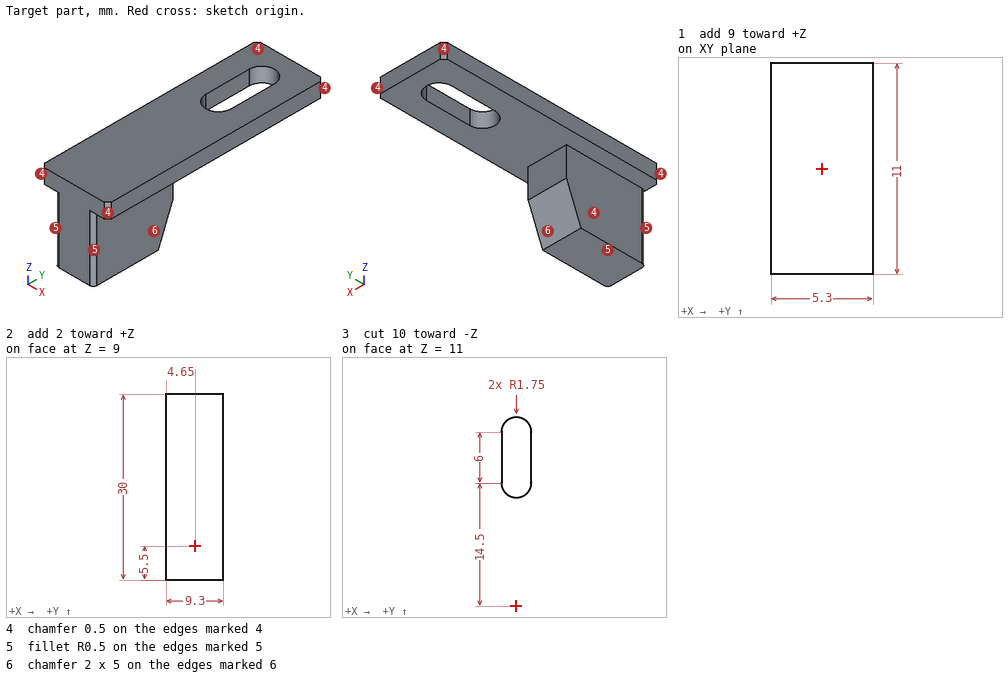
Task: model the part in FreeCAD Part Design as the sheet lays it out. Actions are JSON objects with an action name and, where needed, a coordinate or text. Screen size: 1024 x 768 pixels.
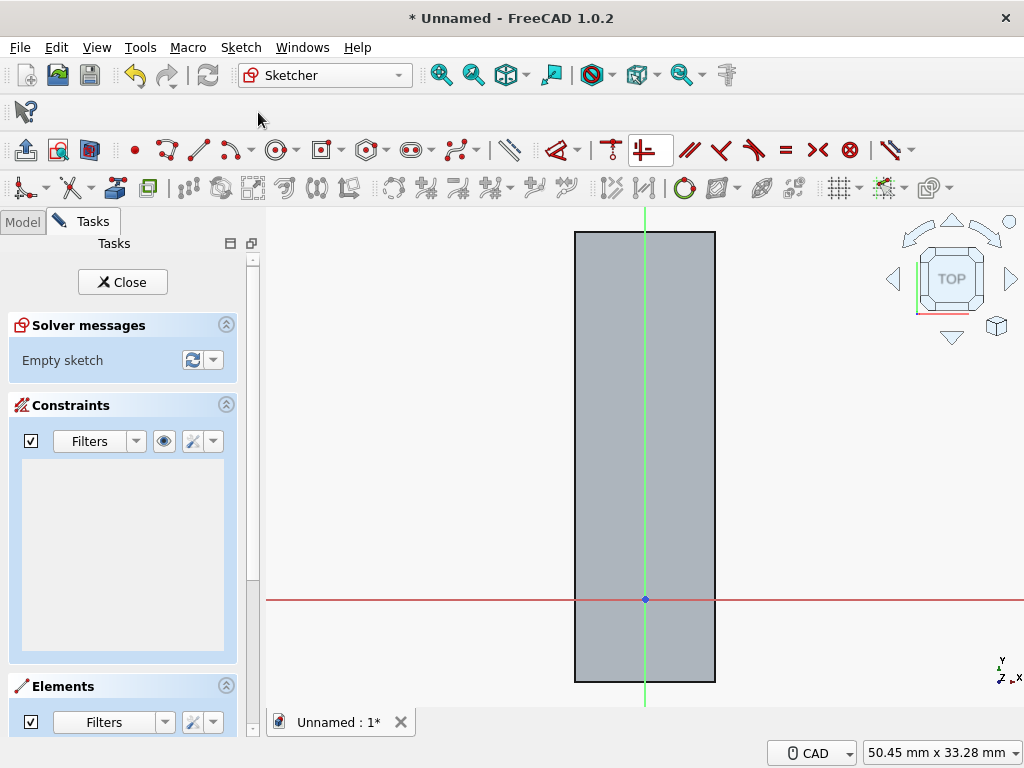
{"action": "left_click", "coordinate": [645, 382]}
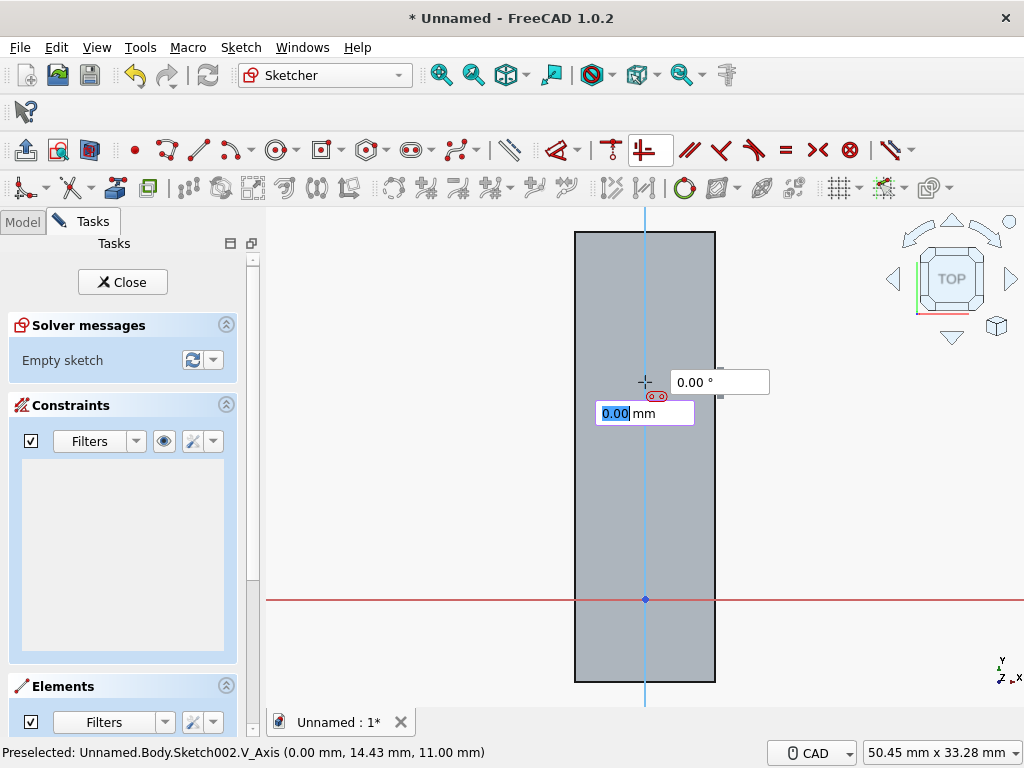
{"action": "left_click", "coordinate": [654, 292]}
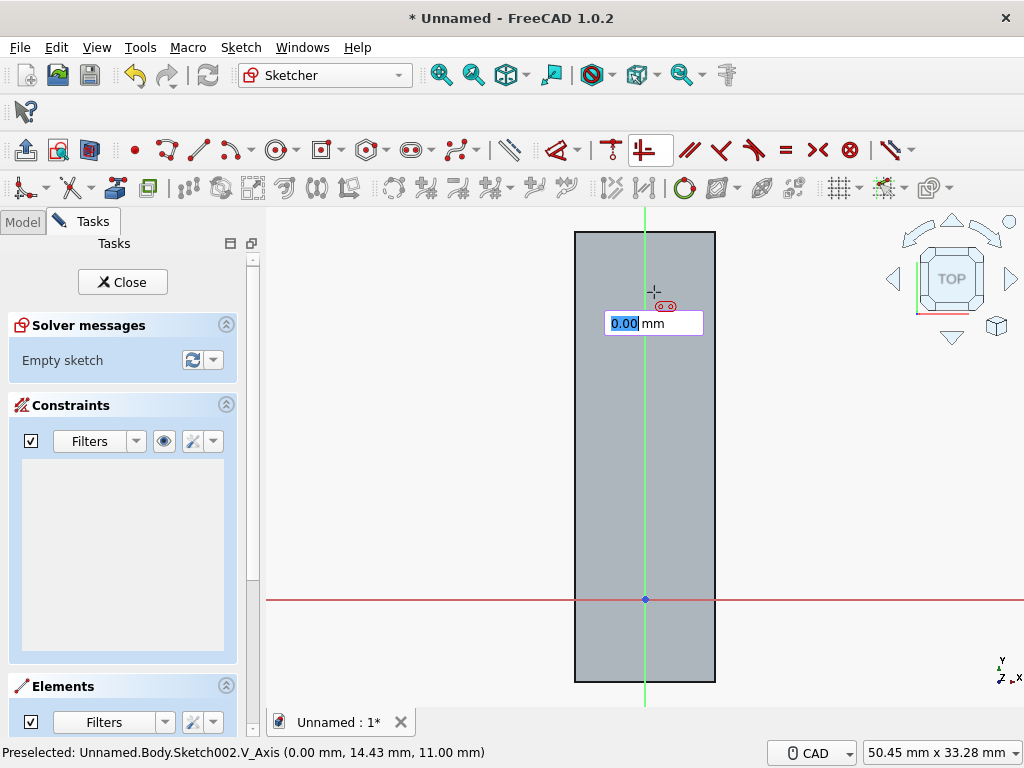
{"action": "left_click", "coordinate": [671, 337]}
{"action": "key", "text": "Escape"}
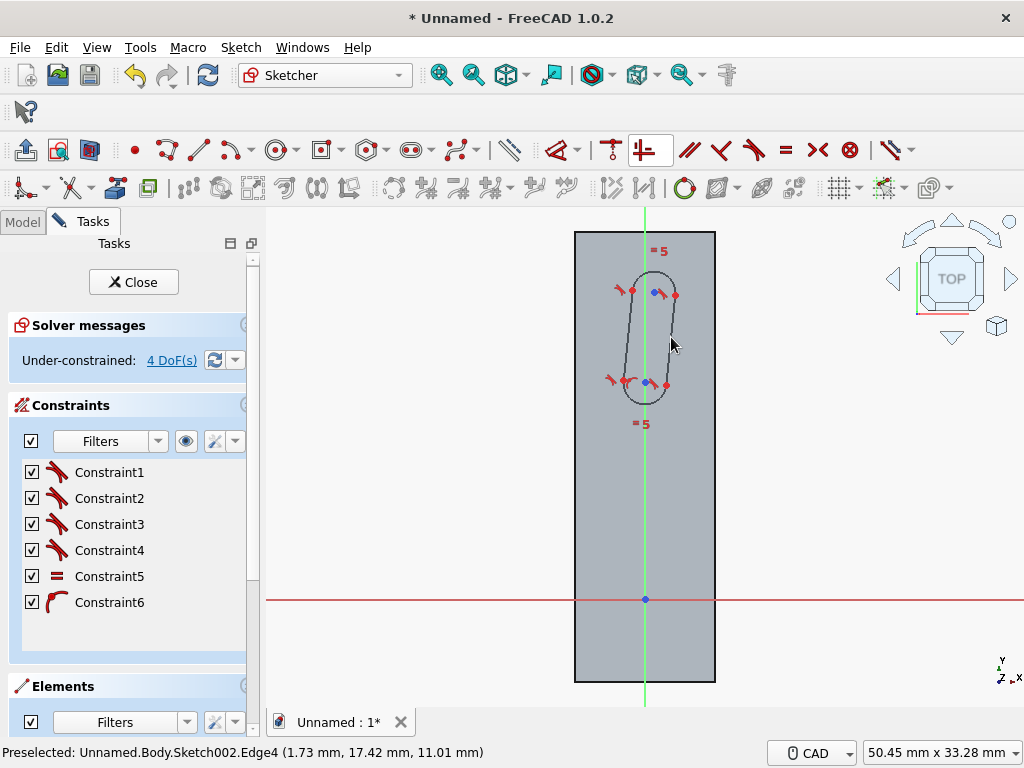
{"action": "left_click", "coordinate": [626, 354]}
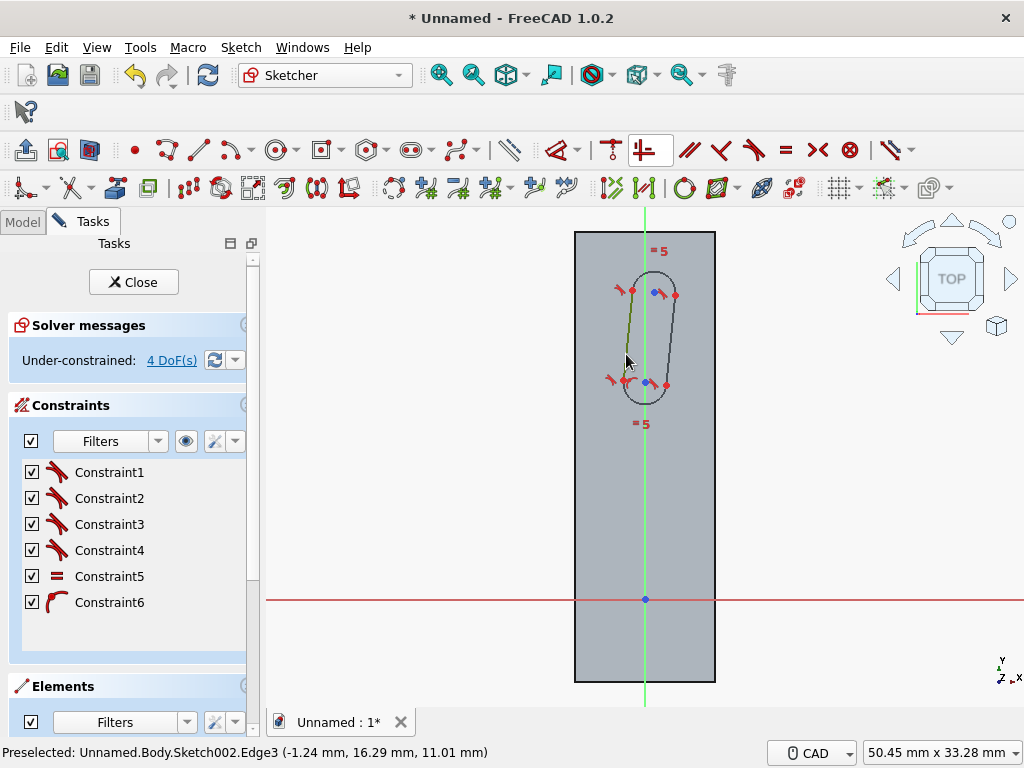
{"action": "key", "text": "v"}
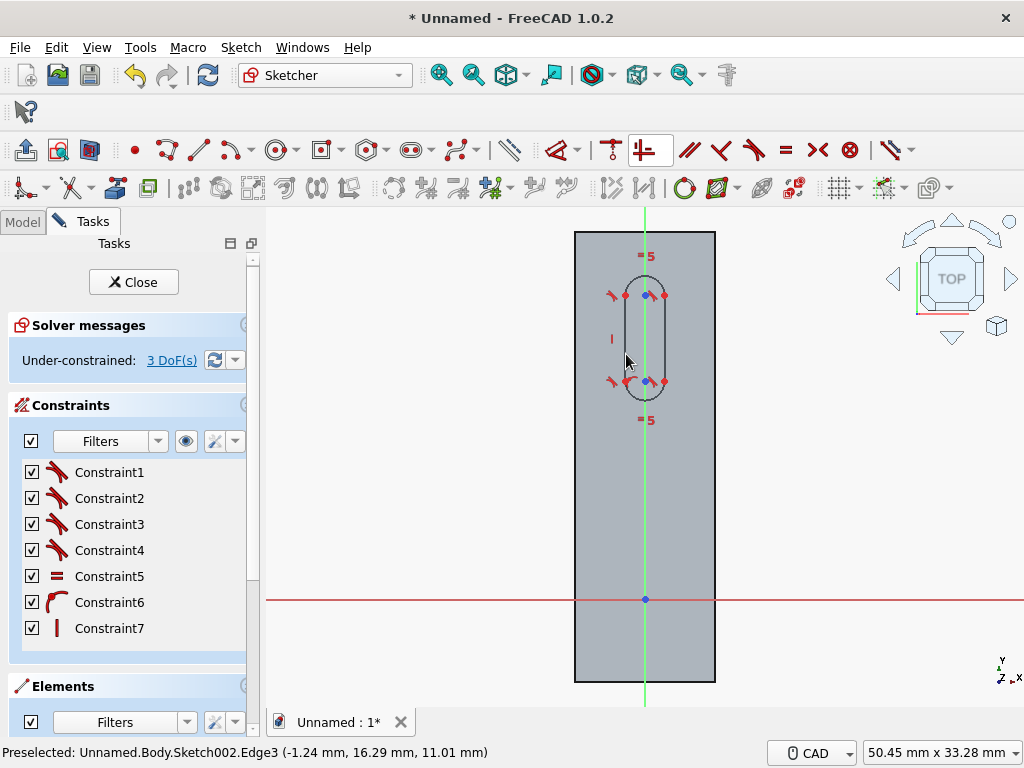
{"action": "left_click", "coordinate": [556, 150]}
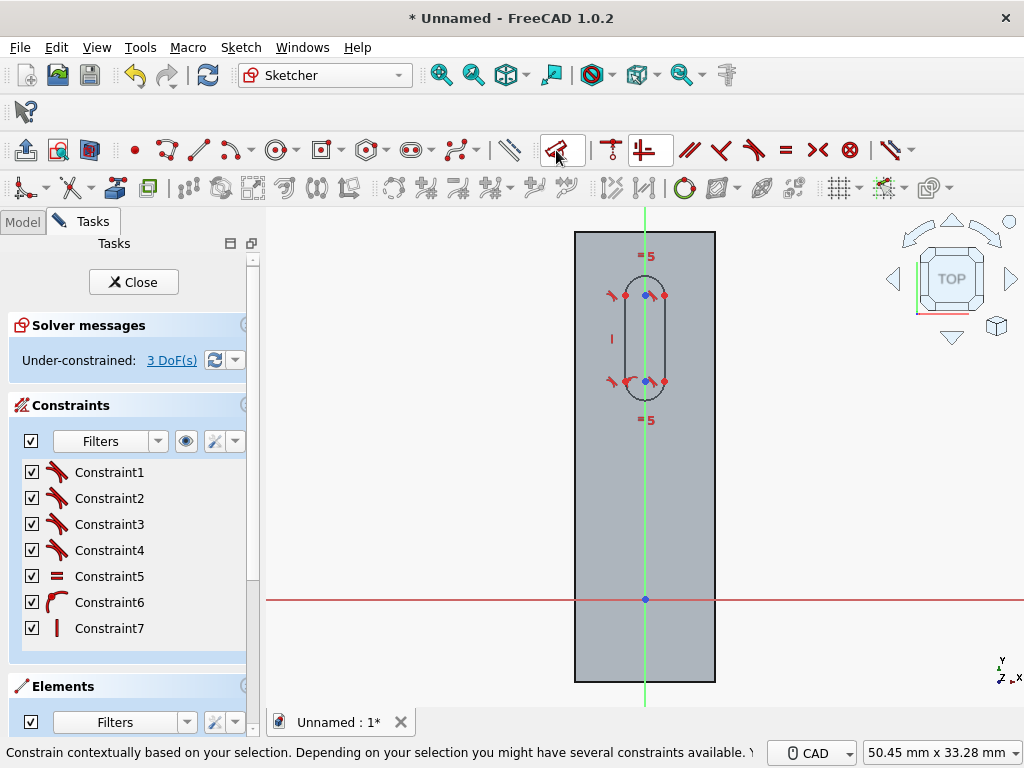
{"action": "scroll", "coordinate": [634, 397], "scroll_direction": "up", "scroll_amount": 3}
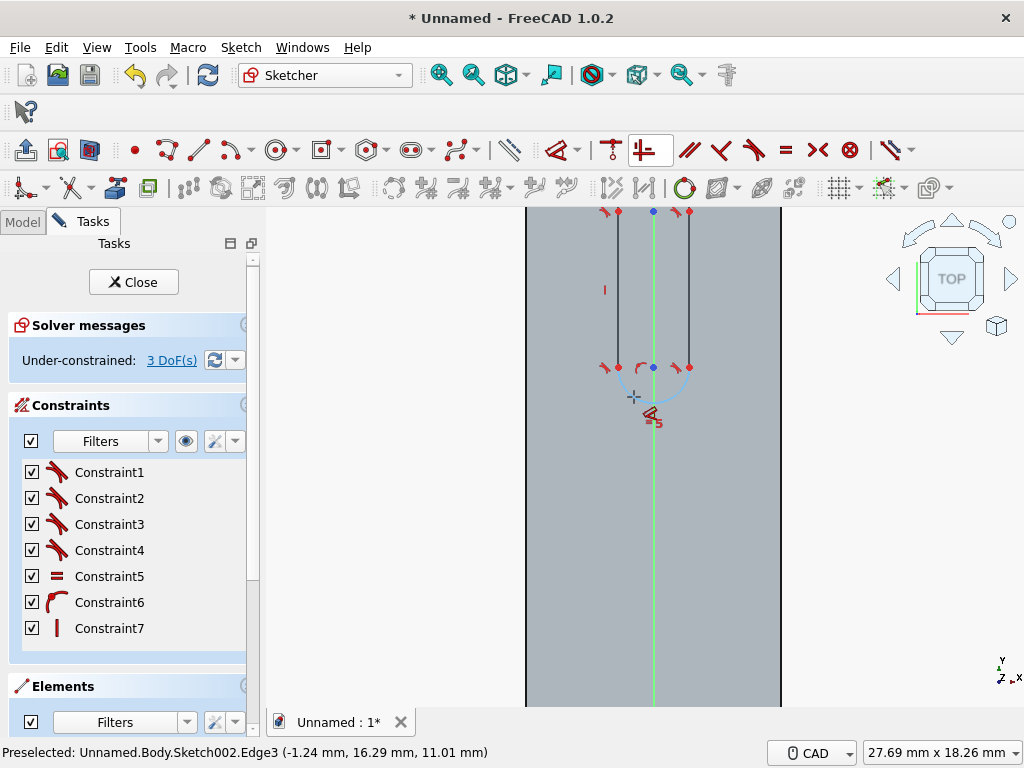
{"action": "left_click", "coordinate": [633, 396]}
{"action": "left_click", "coordinate": [614, 422]}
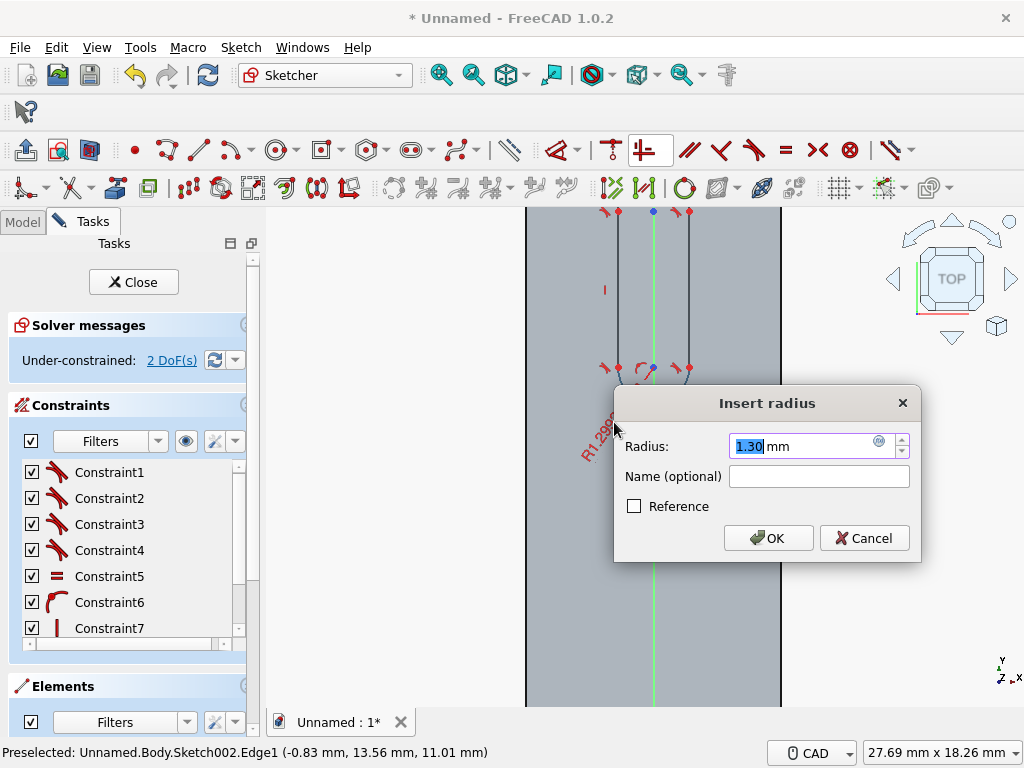
{"action": "type", "text": "1.75"}
{"action": "key", "text": "Return"}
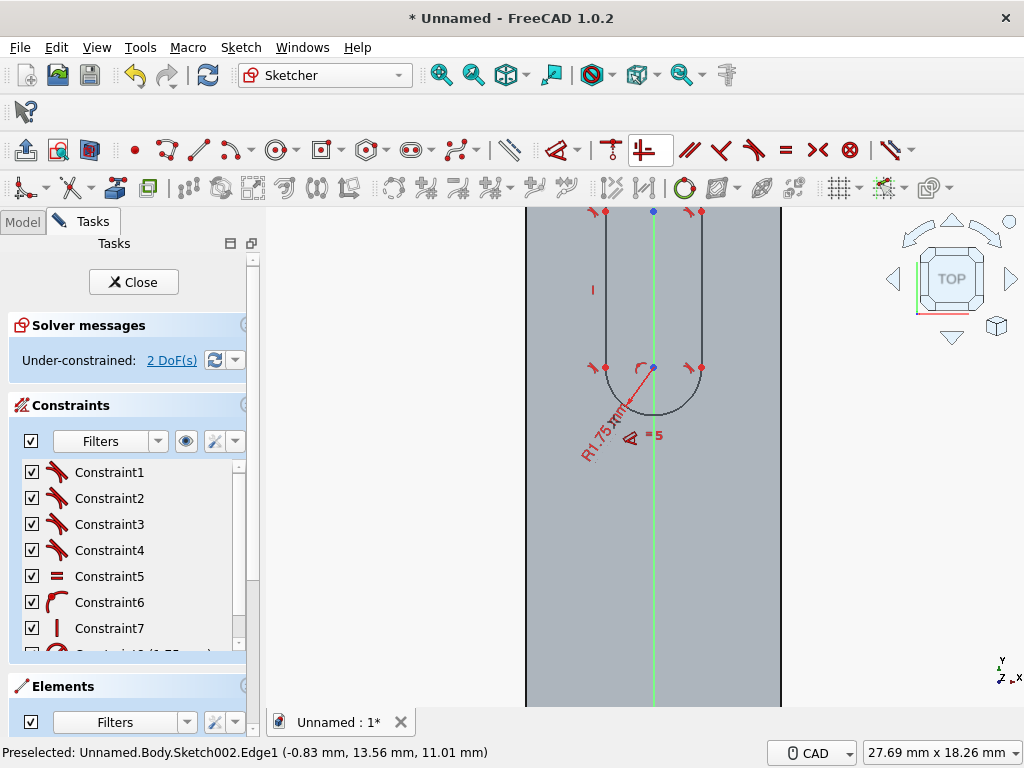
{"action": "left_click", "coordinate": [606, 321]}
{"action": "left_click", "coordinate": [572, 301]}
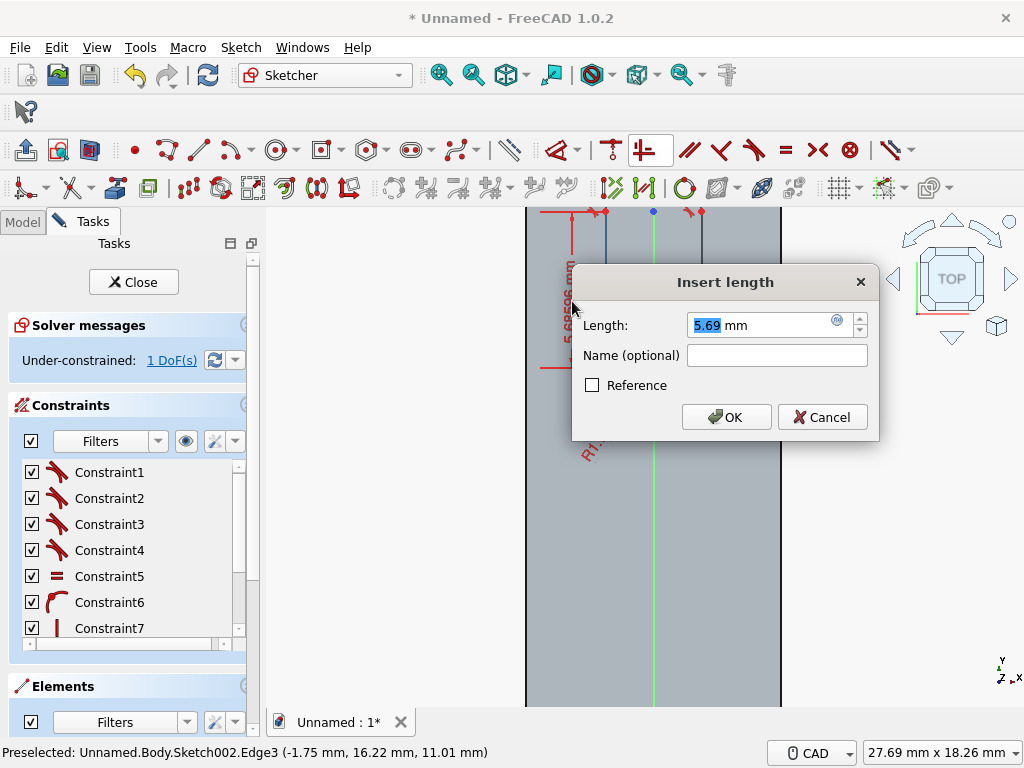
{"action": "type", "text": "6"}
{"action": "key", "text": "Return"}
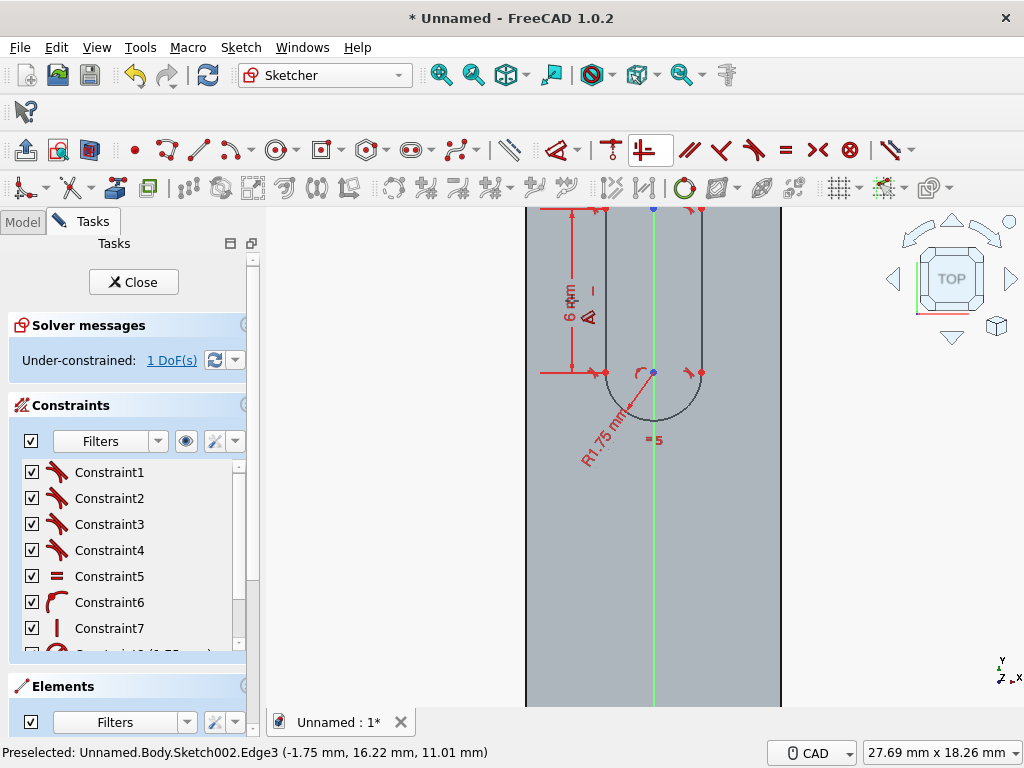
{"action": "left_click", "coordinate": [606, 373]}
{"action": "left_click", "coordinate": [572, 526]}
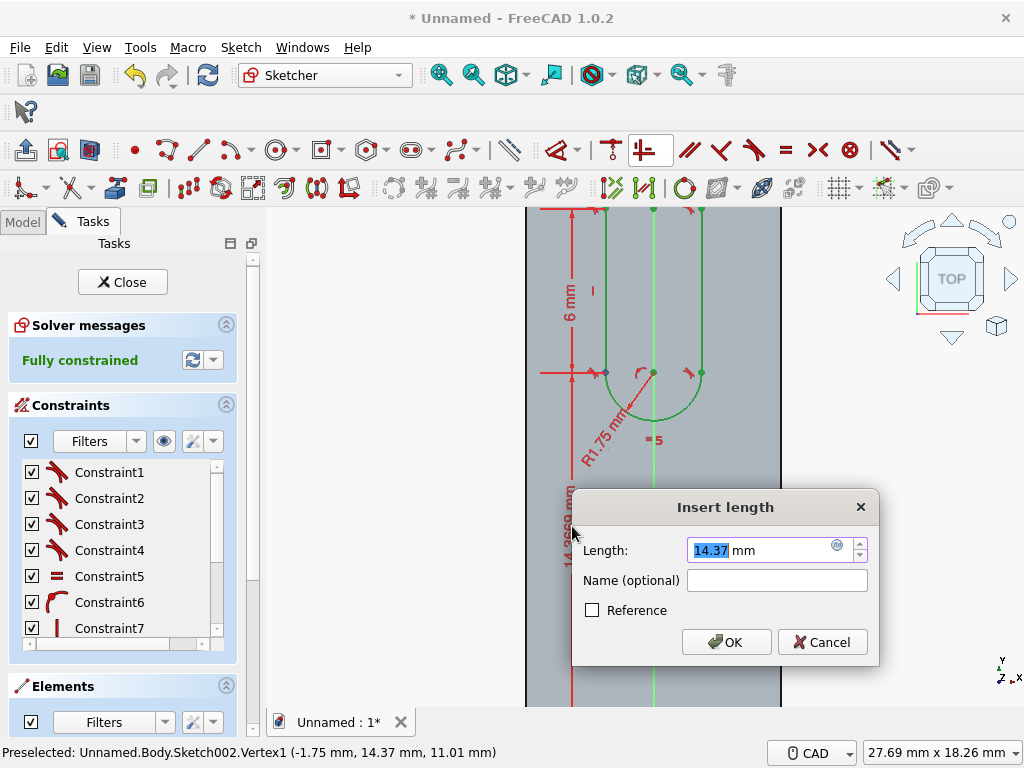
{"action": "type", "text": "14.5"}
{"action": "key", "text": "Return"}
{"action": "key", "text": "Escape"}